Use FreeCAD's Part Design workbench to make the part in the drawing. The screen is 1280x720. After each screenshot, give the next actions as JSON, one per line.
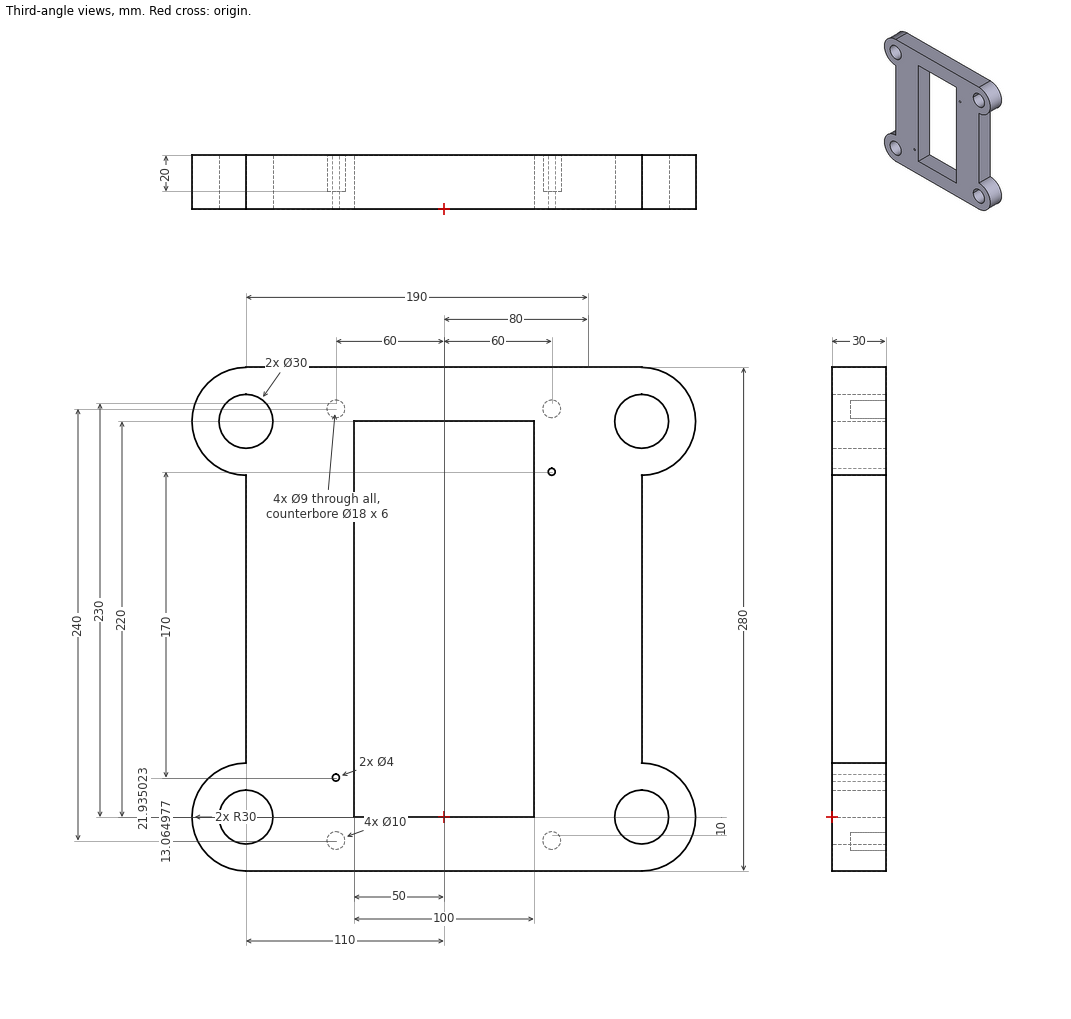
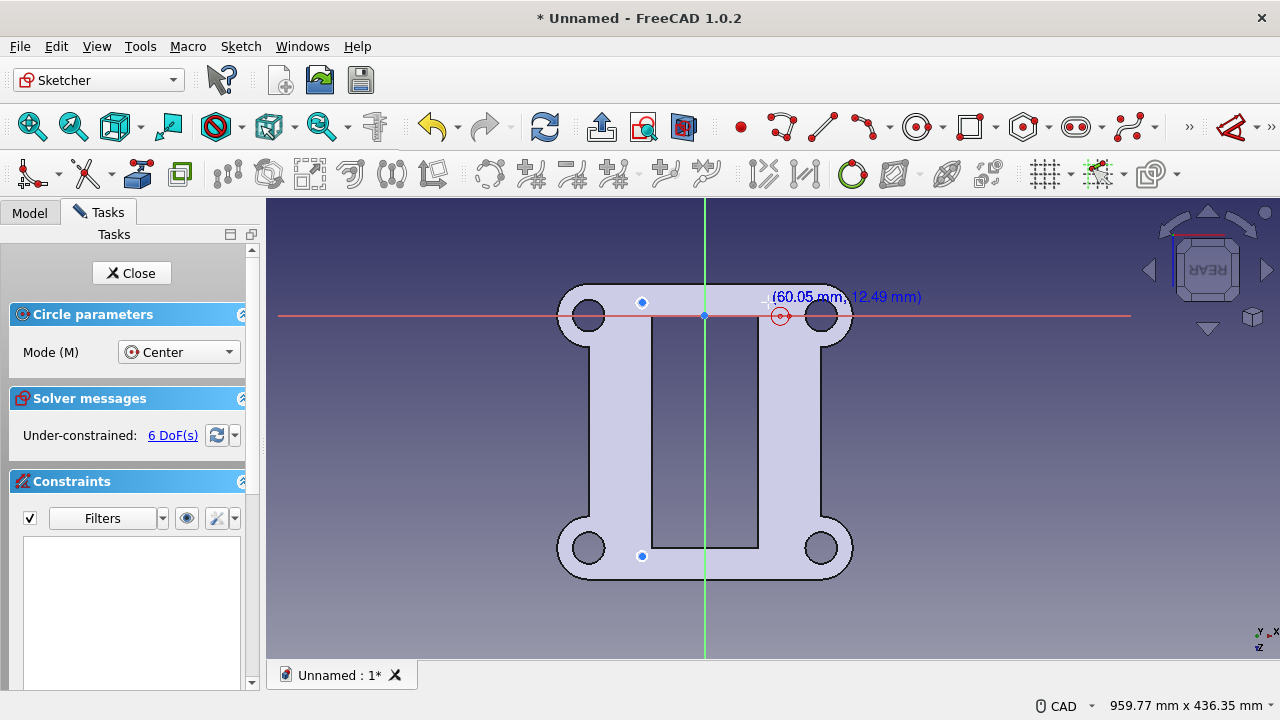
{"action": "left_click", "coordinate": [768, 302]}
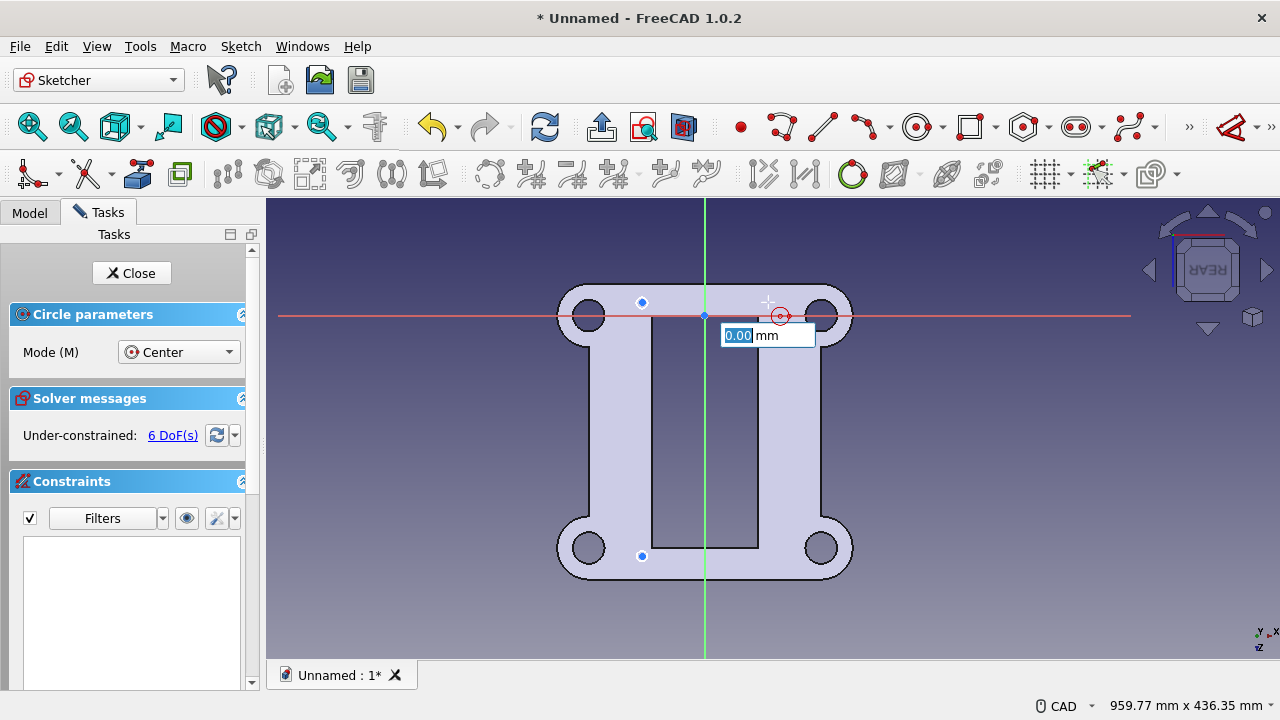
{"action": "scroll", "coordinate": [772, 298], "scroll_direction": "up", "scroll_amount": 6}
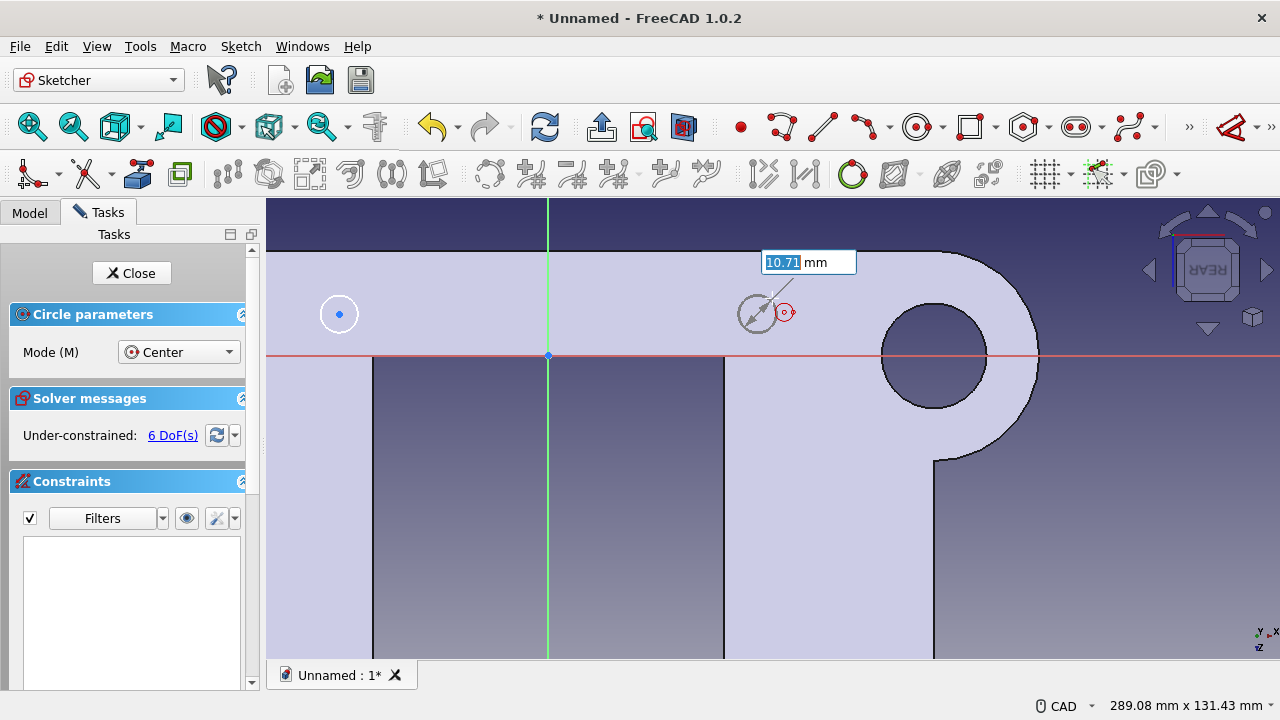
{"action": "left_click", "coordinate": [771, 298]}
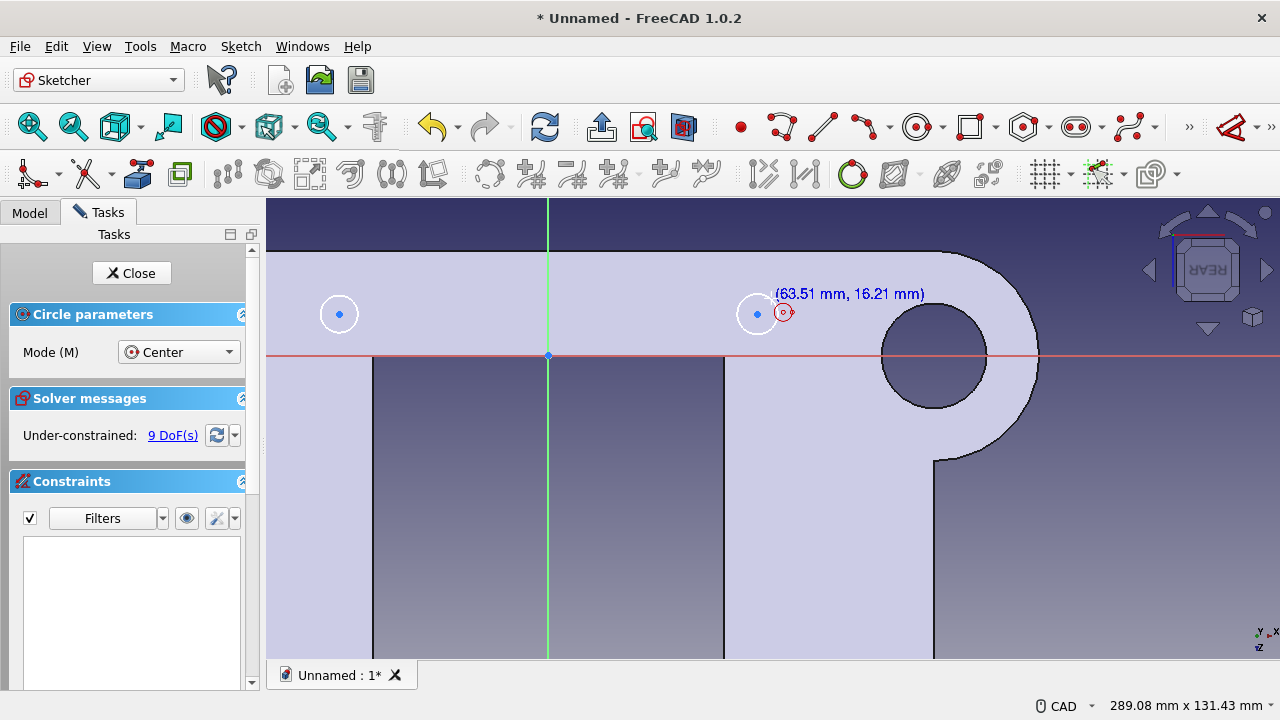
{"action": "scroll", "coordinate": [772, 298], "scroll_direction": "down", "scroll_amount": 6}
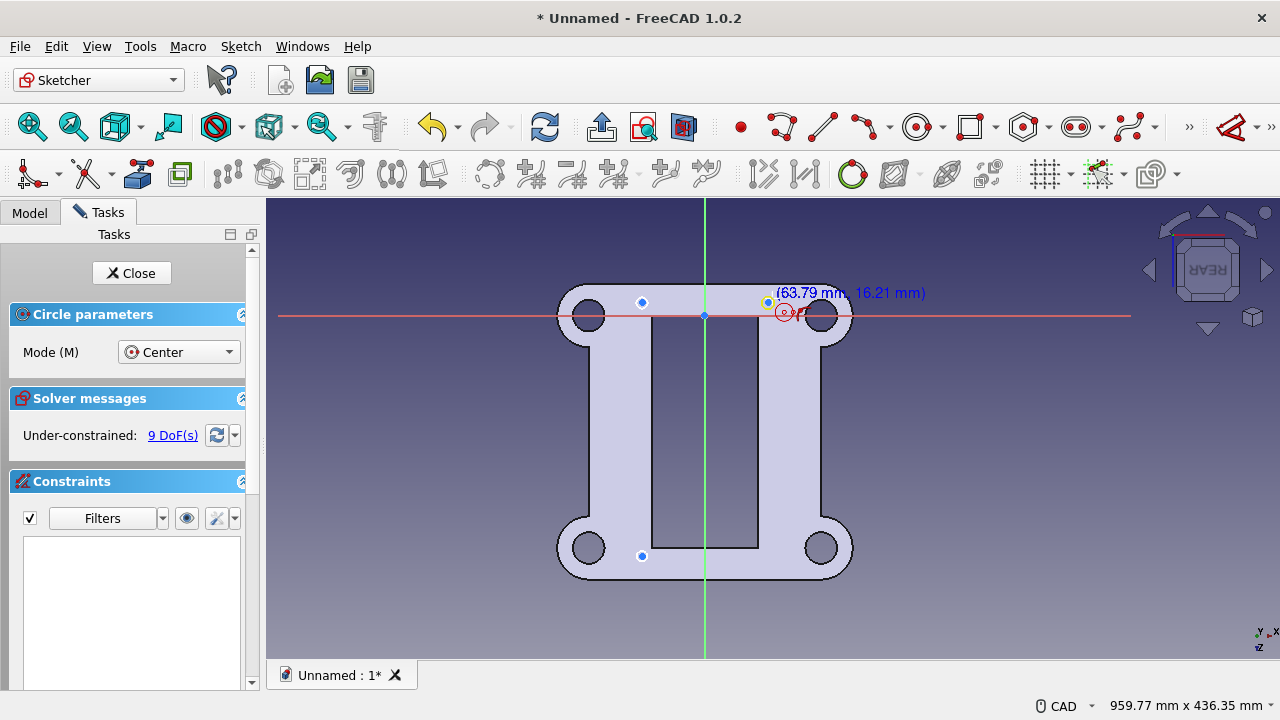
{"action": "scroll", "coordinate": [768, 555], "scroll_direction": "up", "scroll_amount": 8}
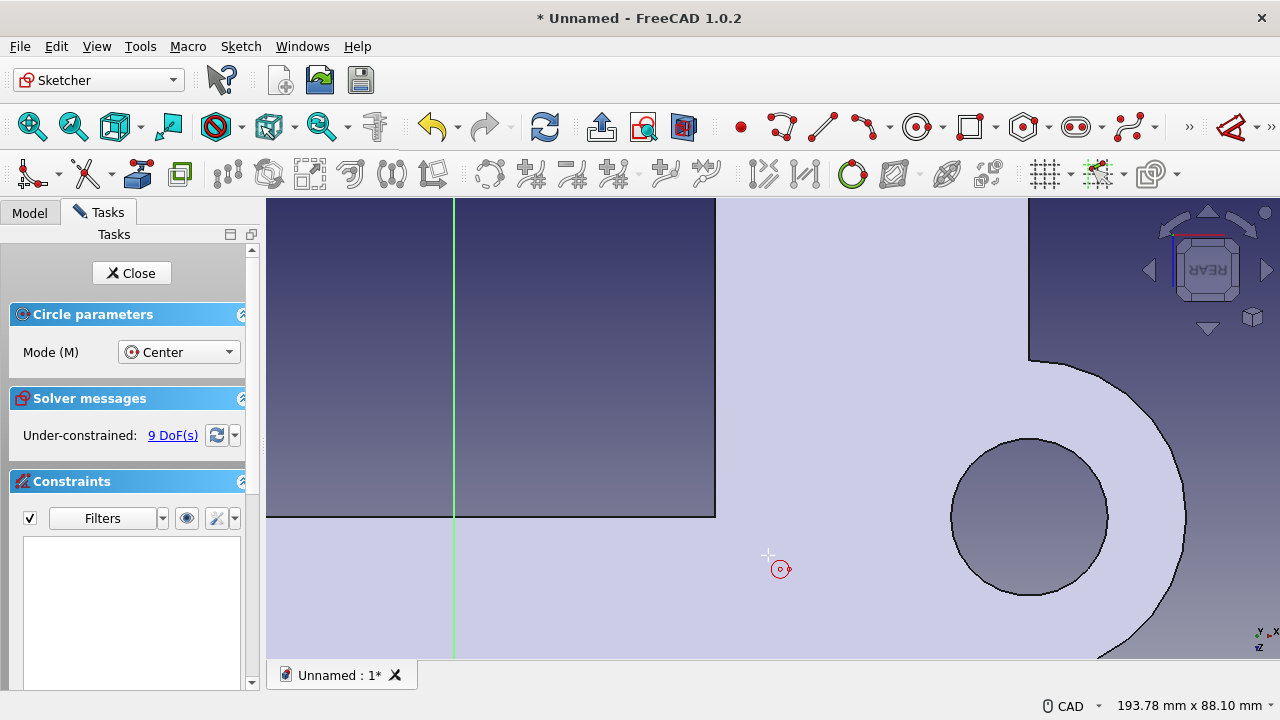
{"action": "scroll", "coordinate": [768, 556], "scroll_direction": "down", "scroll_amount": 8}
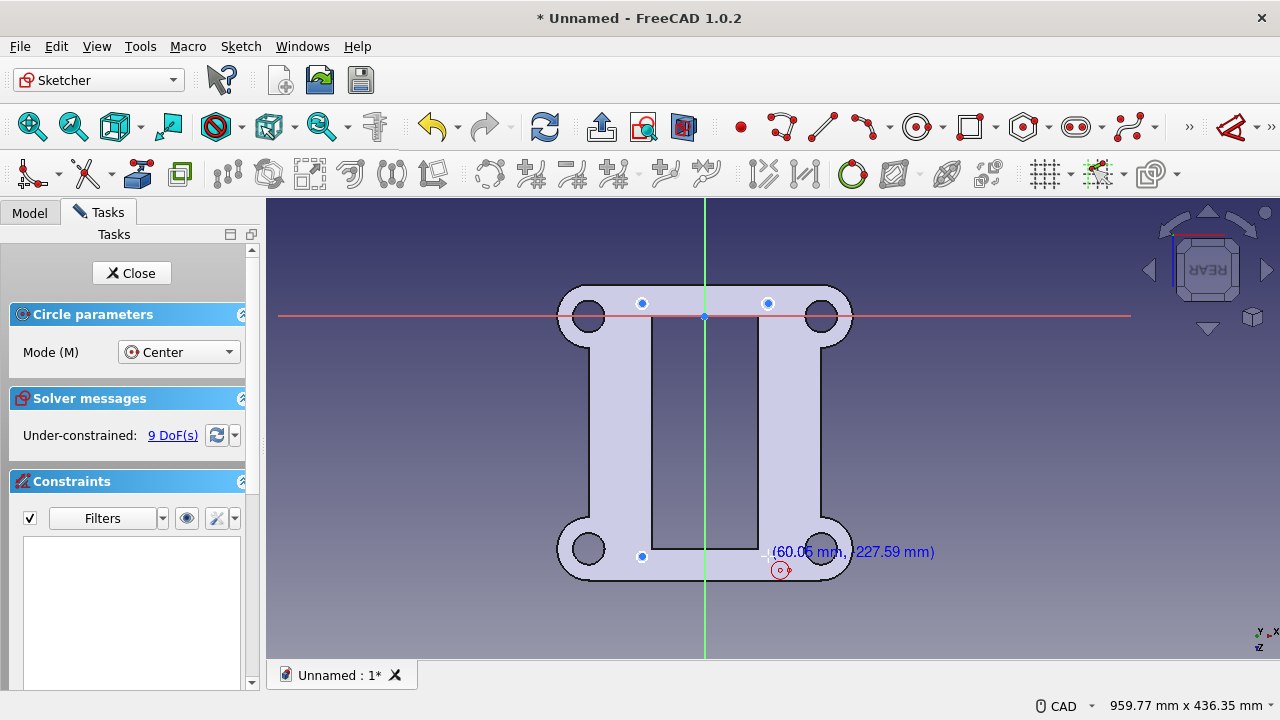
{"action": "left_click", "coordinate": [768, 556]}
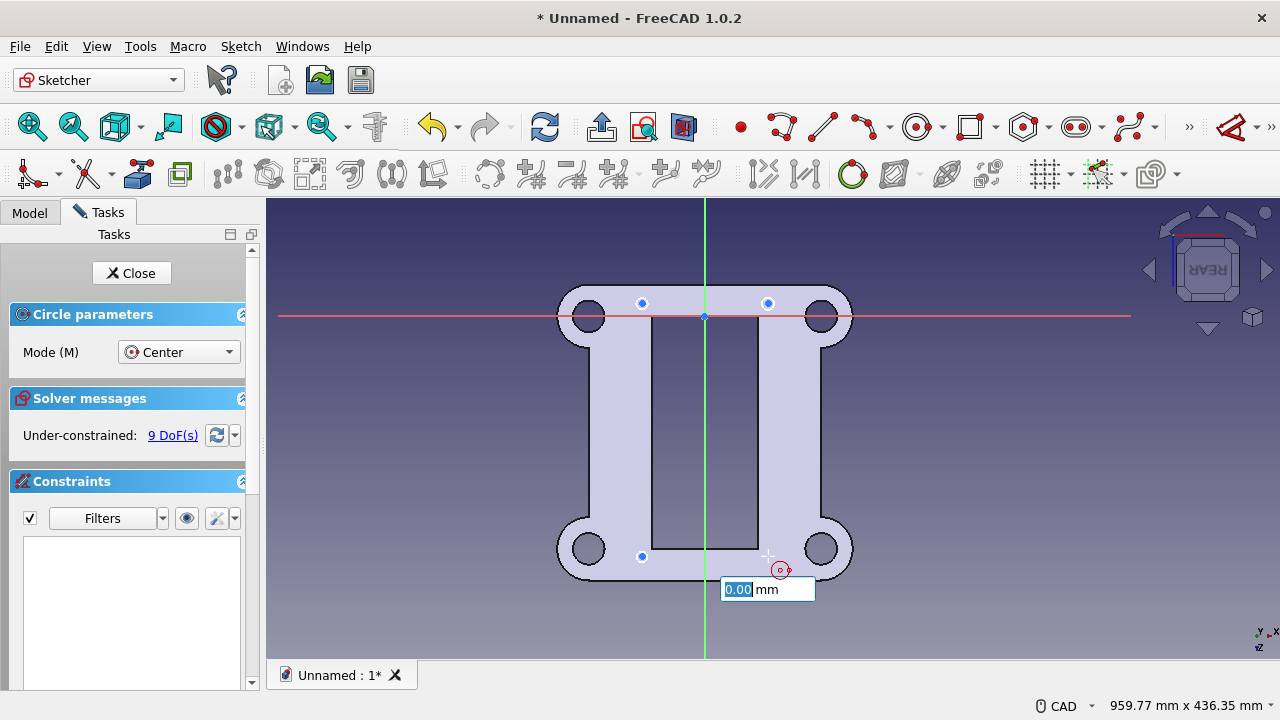
{"action": "scroll", "coordinate": [772, 552], "scroll_direction": "up", "scroll_amount": 6}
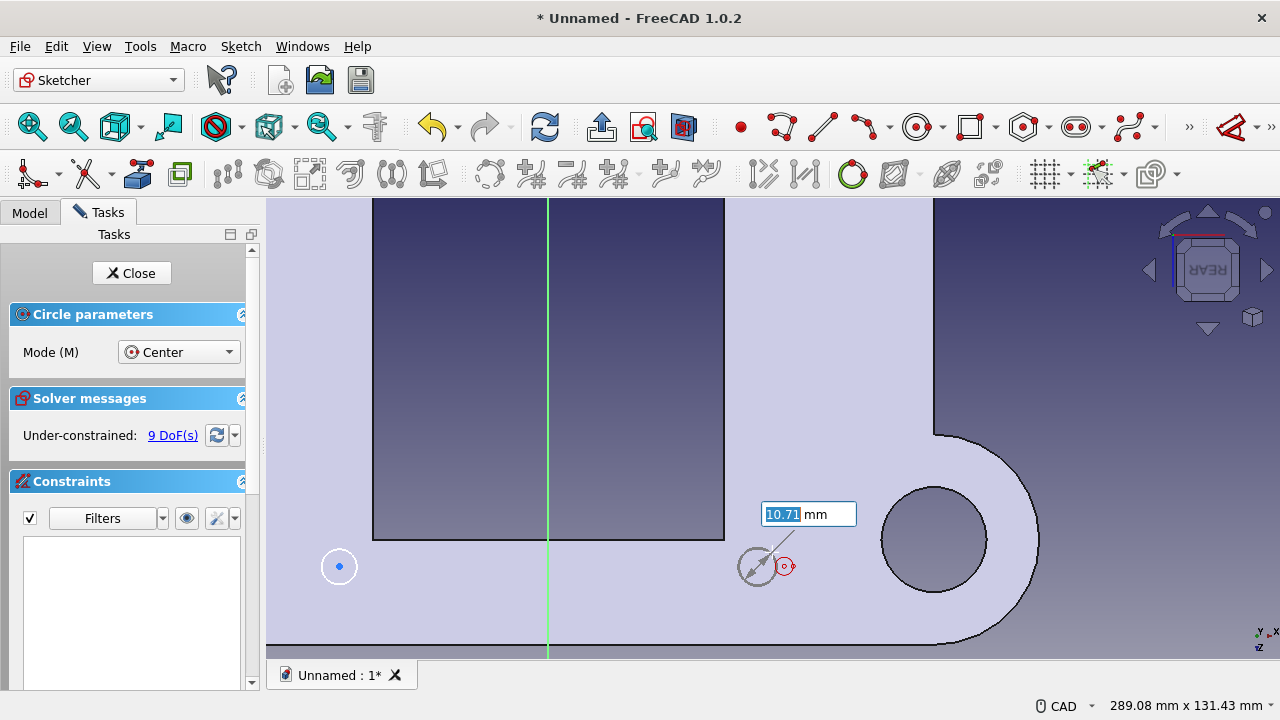
{"action": "left_click", "coordinate": [771, 552]}
{"action": "key", "text": "Escape"}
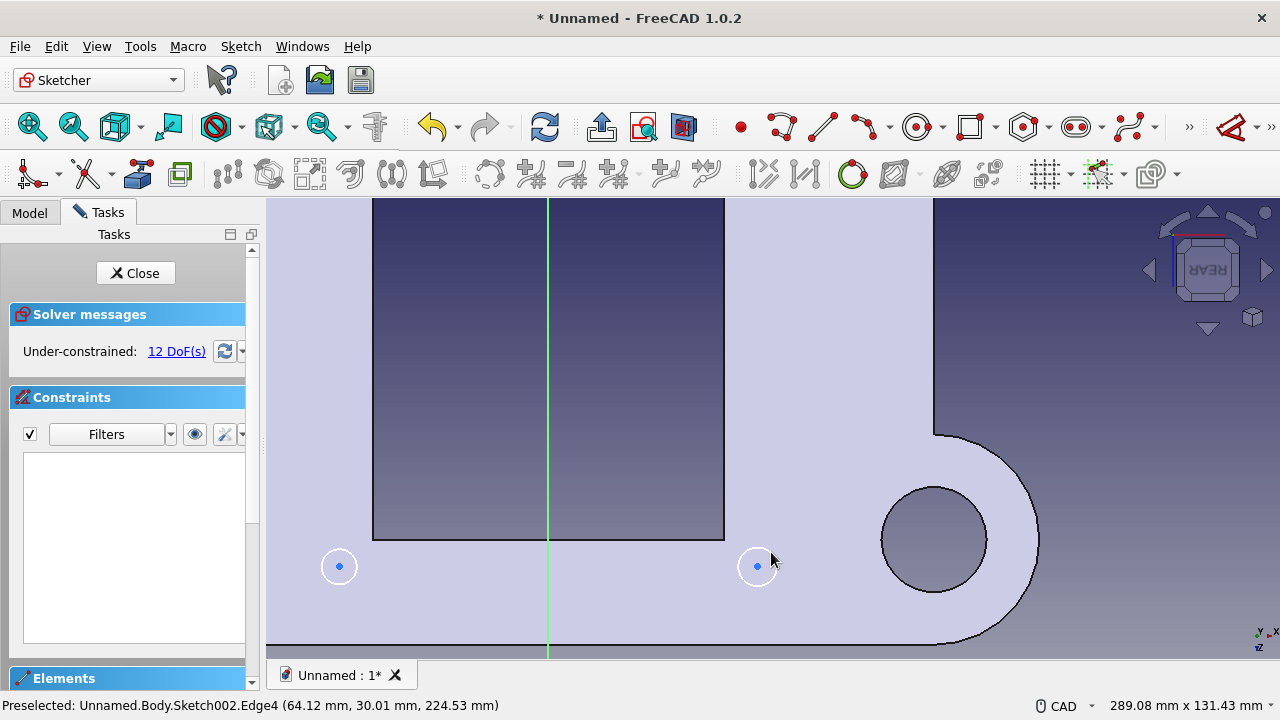
{"action": "scroll", "coordinate": [772, 552], "scroll_direction": "down", "scroll_amount": 6}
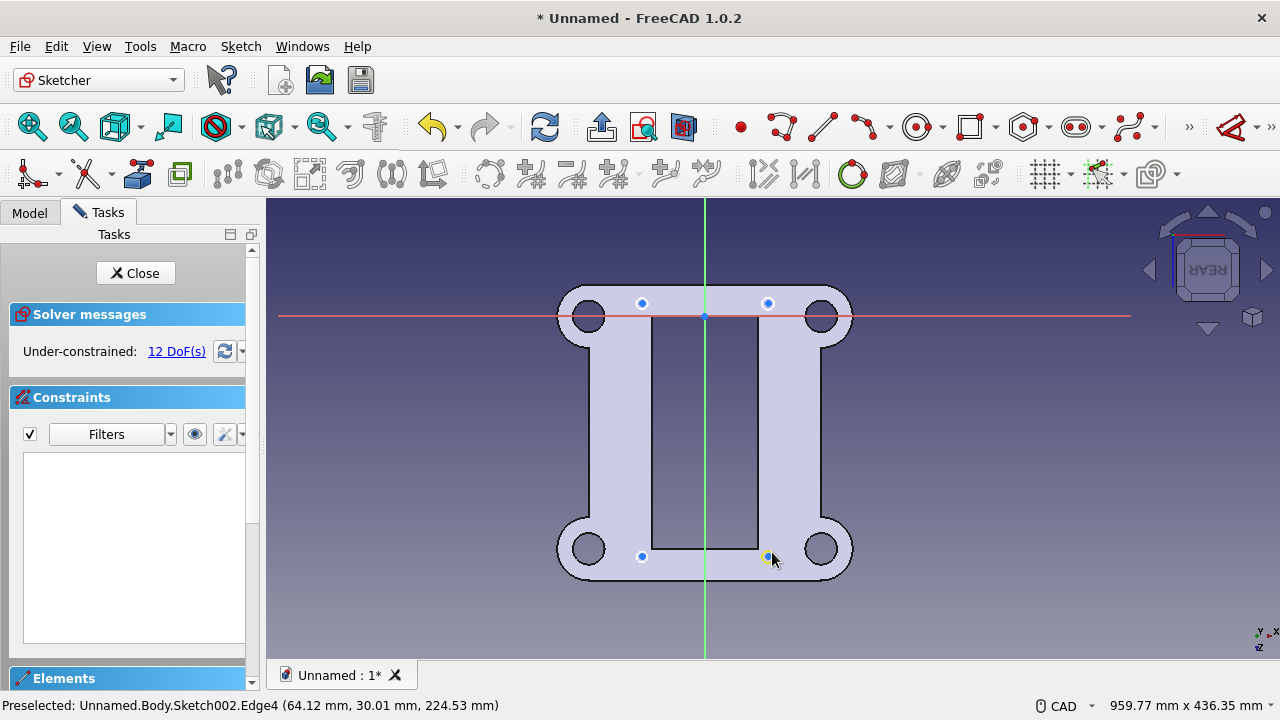
{"action": "scroll", "coordinate": [646, 300], "scroll_direction": "up", "scroll_amount": 5}